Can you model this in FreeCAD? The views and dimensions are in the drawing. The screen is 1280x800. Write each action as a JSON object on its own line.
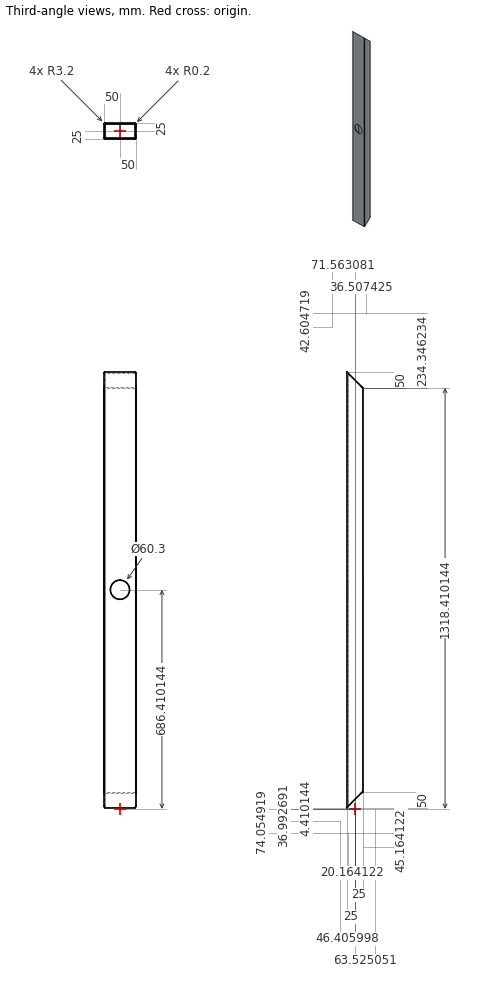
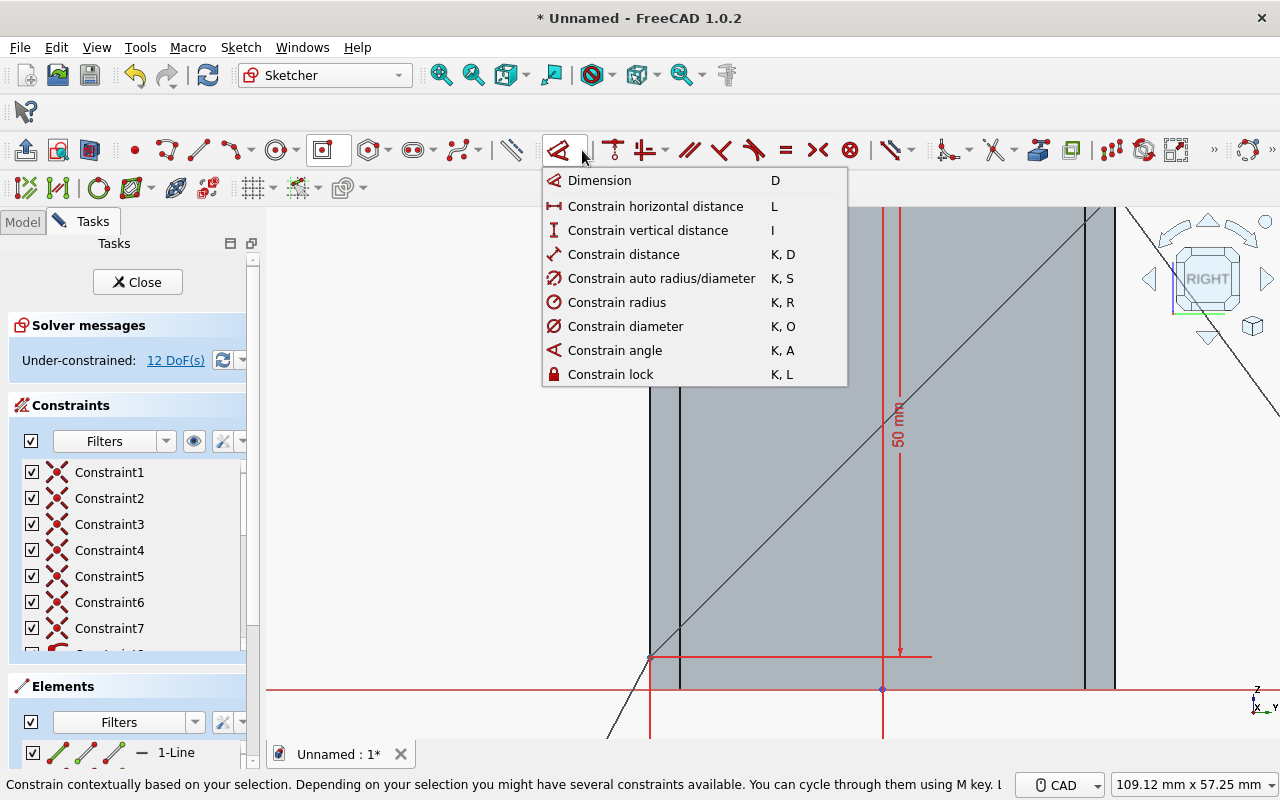
{"action": "left_click", "coordinate": [695, 230]}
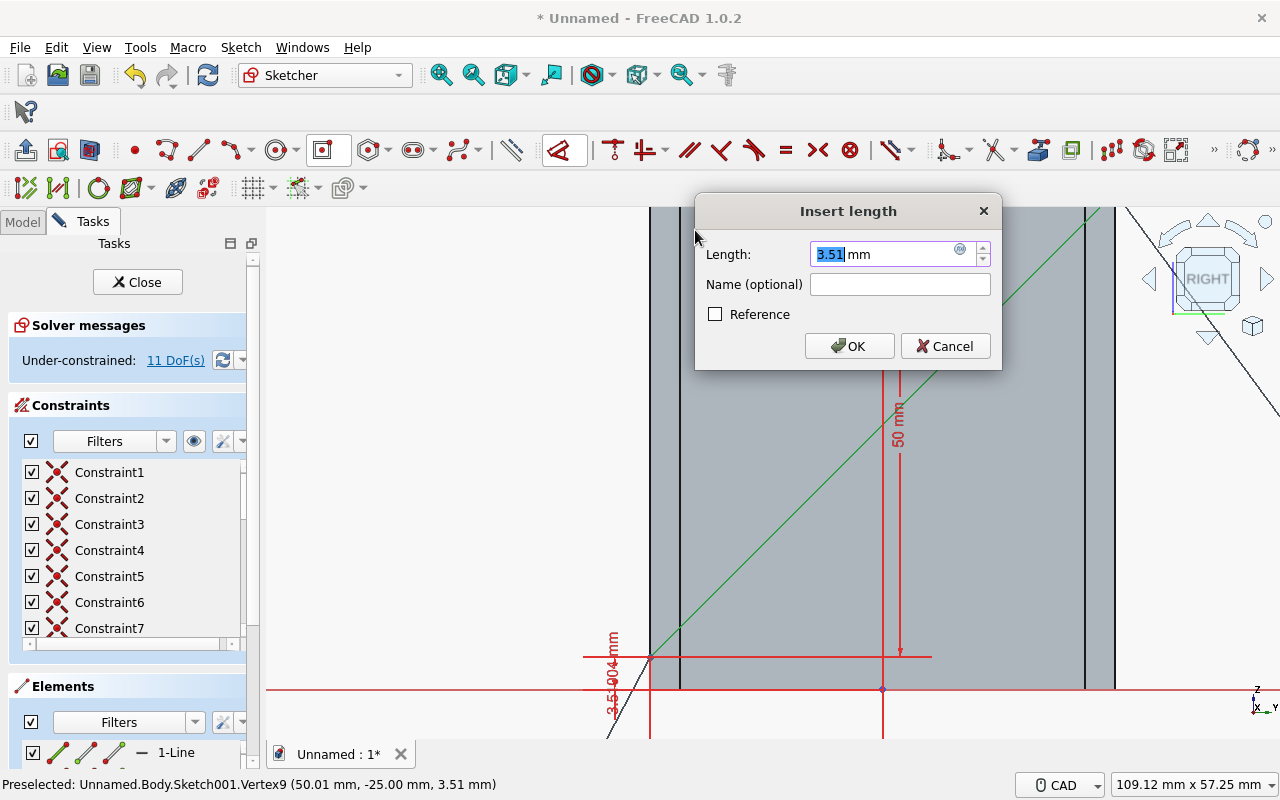
{"action": "type", "text": "4.410144"}
{"action": "key", "text": "Return"}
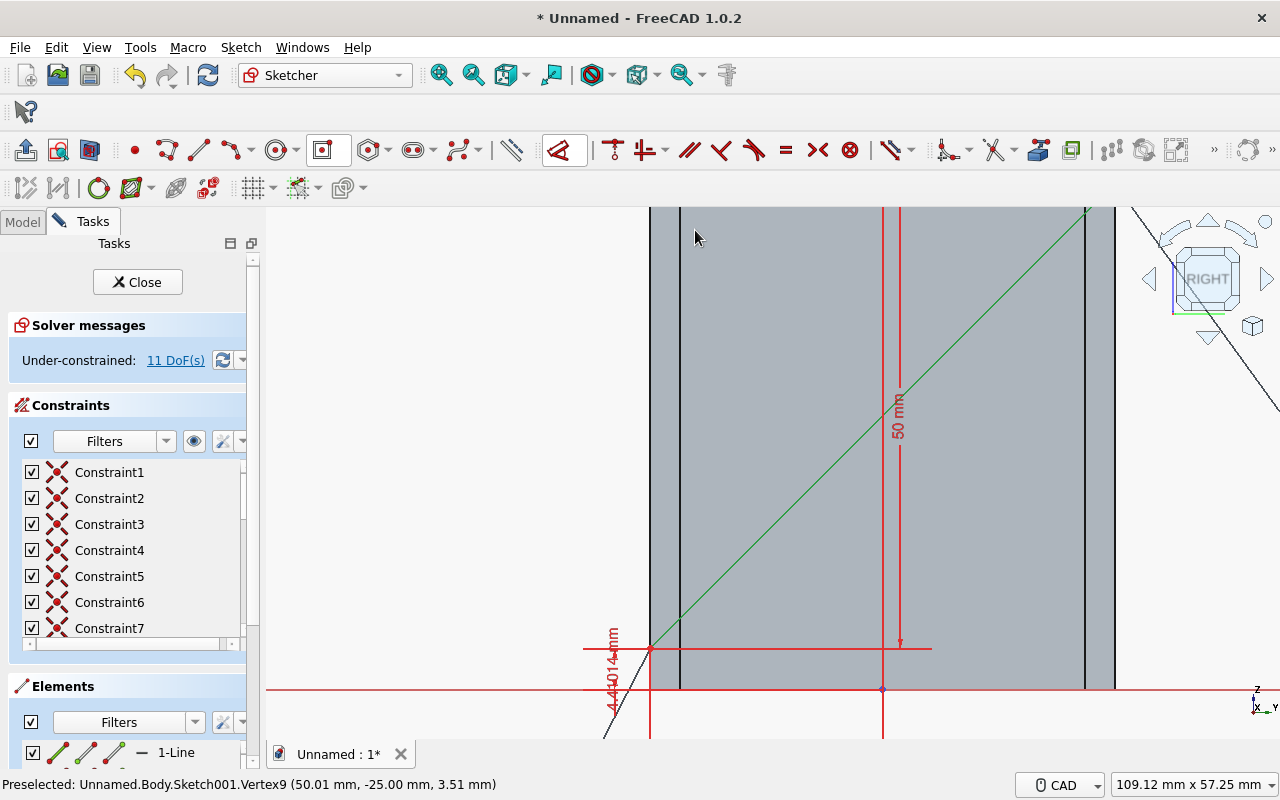
{"action": "scroll", "coordinate": [701, 654], "scroll_direction": "down", "scroll_amount": 18}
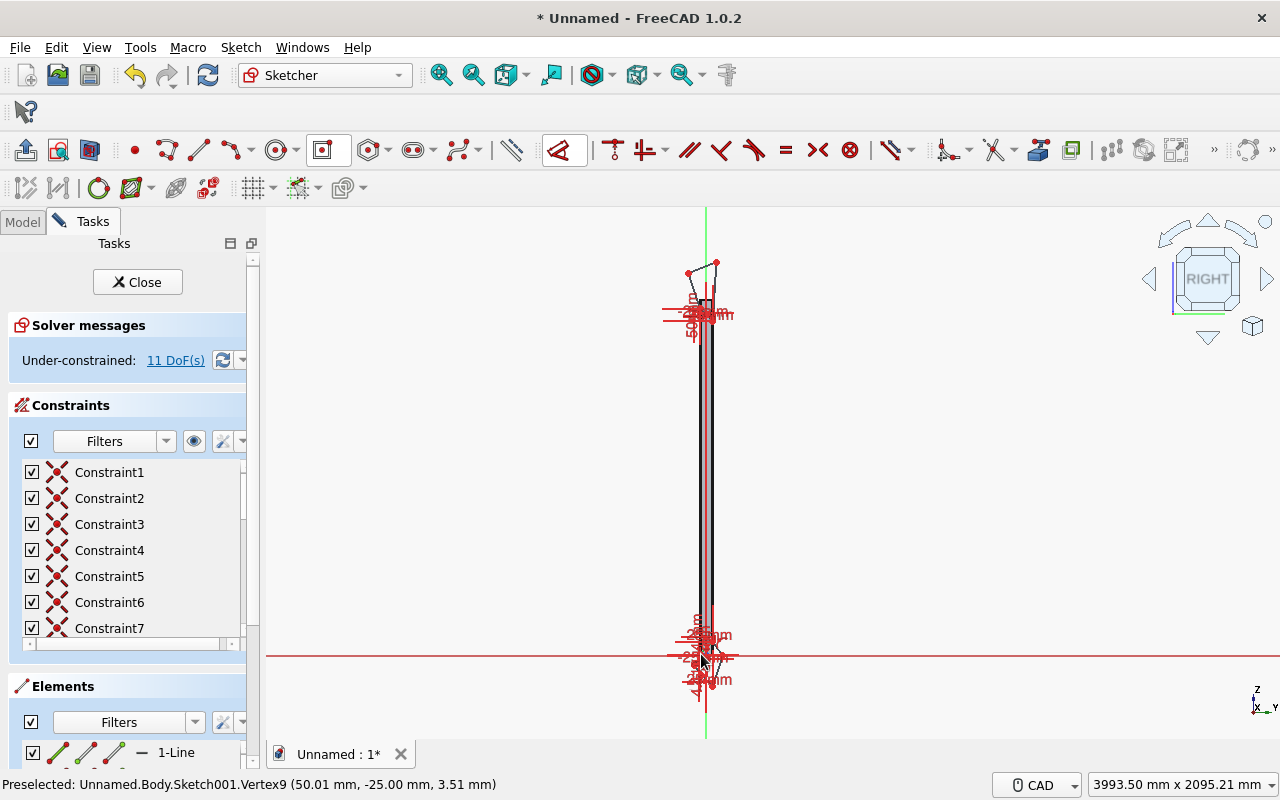
{"action": "scroll", "coordinate": [701, 469], "scroll_direction": "down", "scroll_amount": 1}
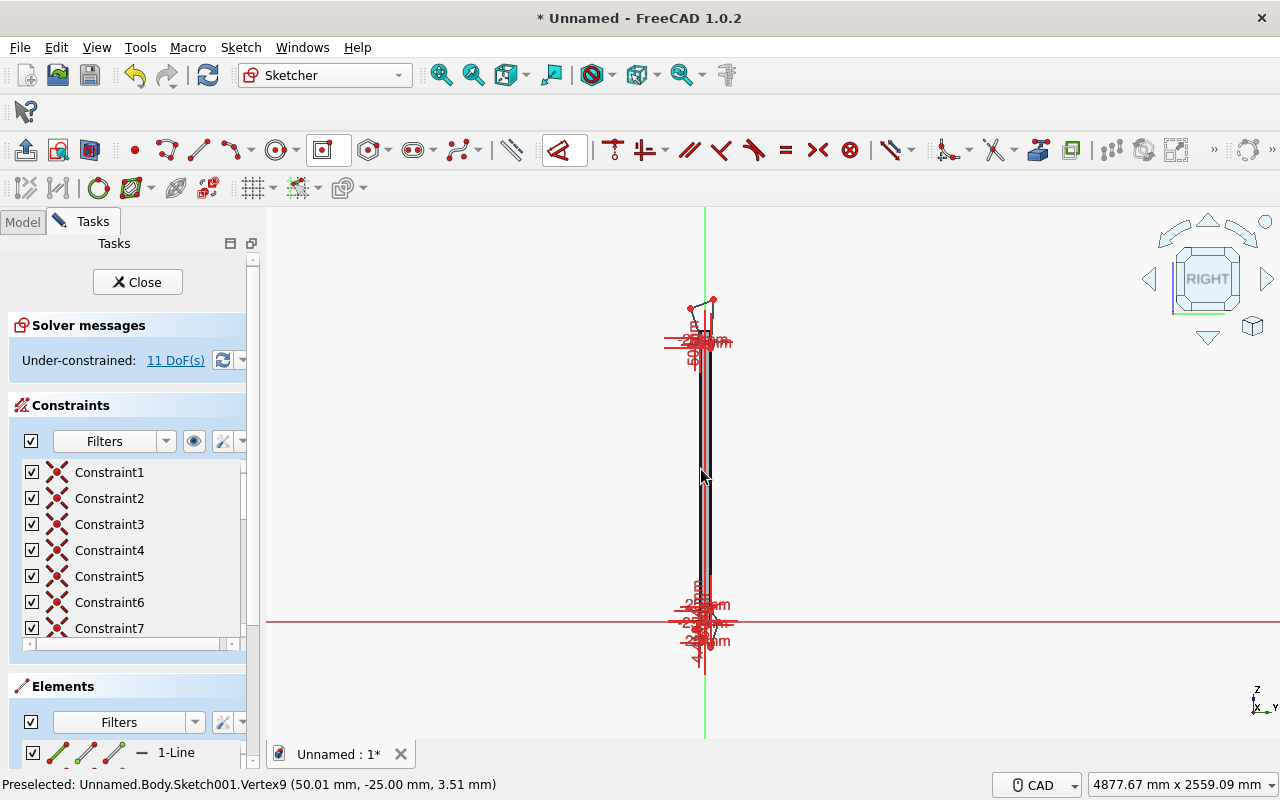
{"action": "scroll", "coordinate": [714, 300], "scroll_direction": "up", "scroll_amount": 9}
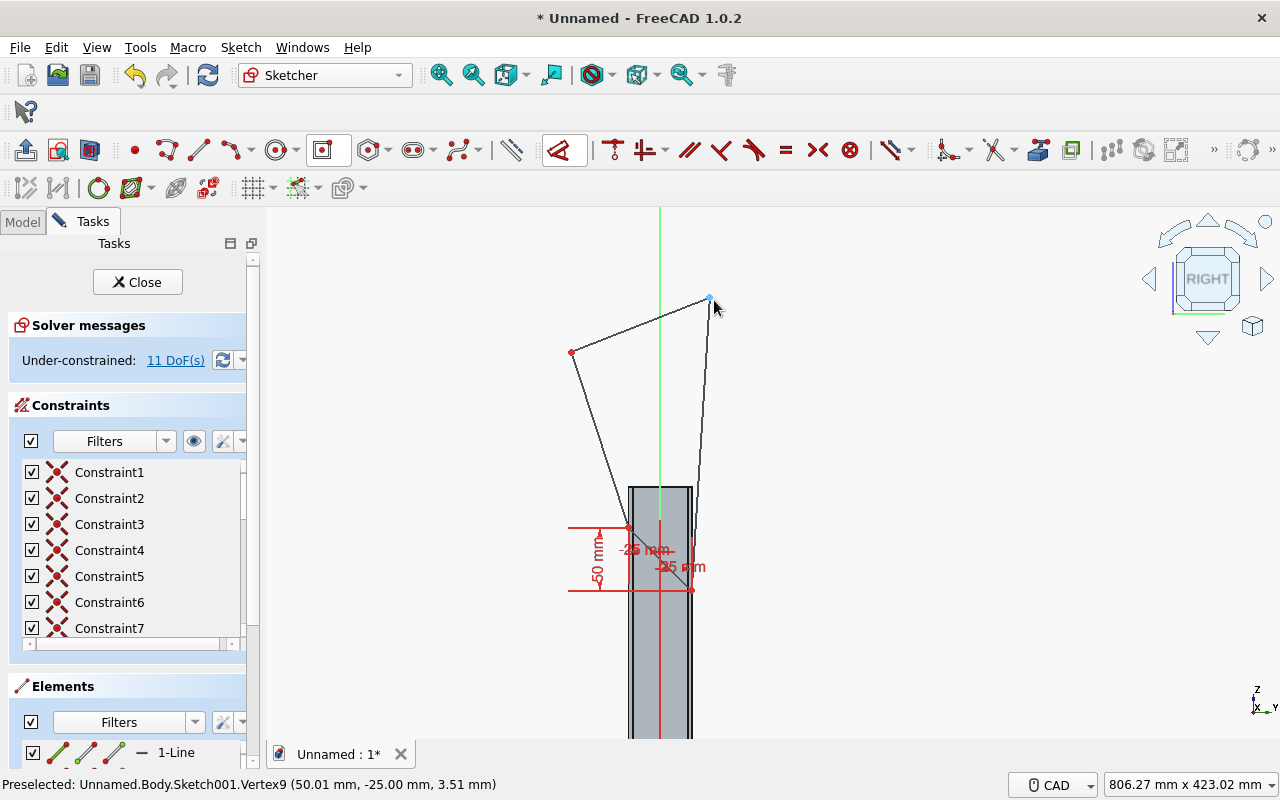
{"action": "left_click", "coordinate": [710, 298]}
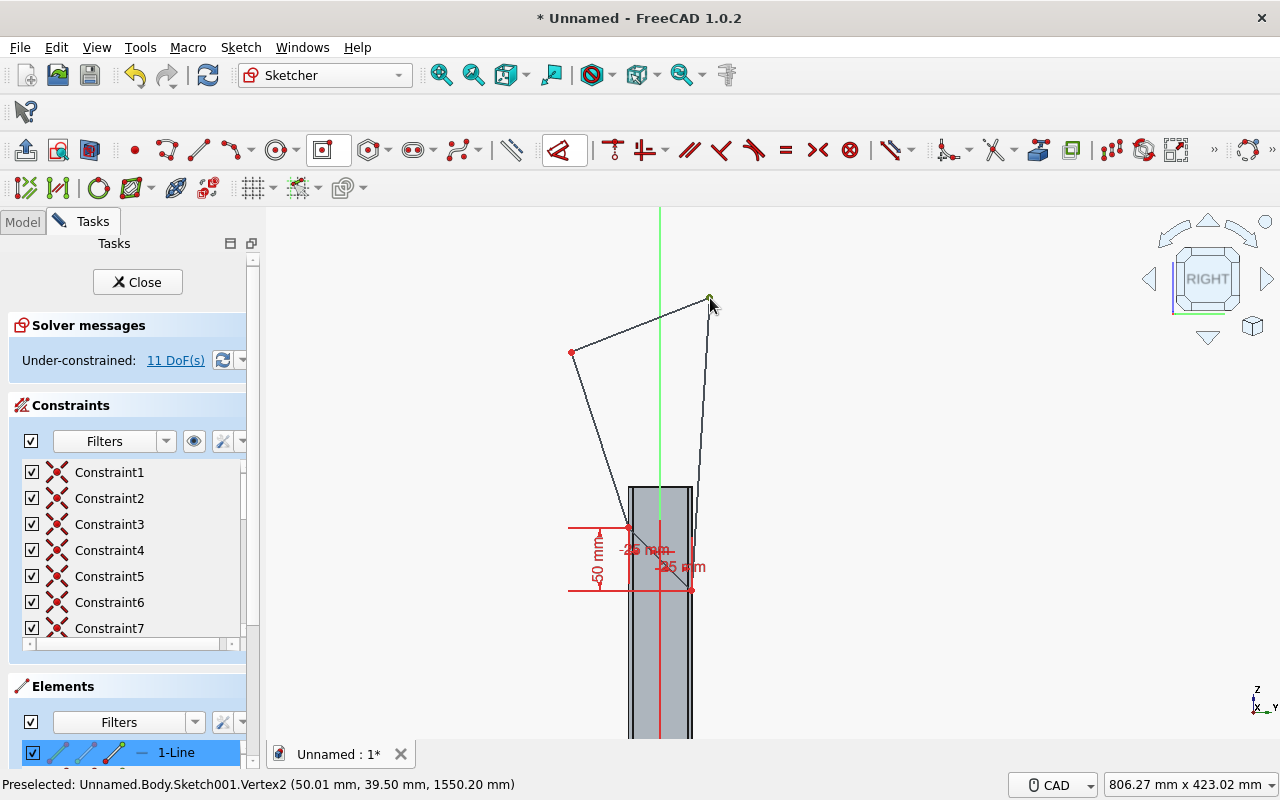
{"action": "left_click", "coordinate": [582, 150]}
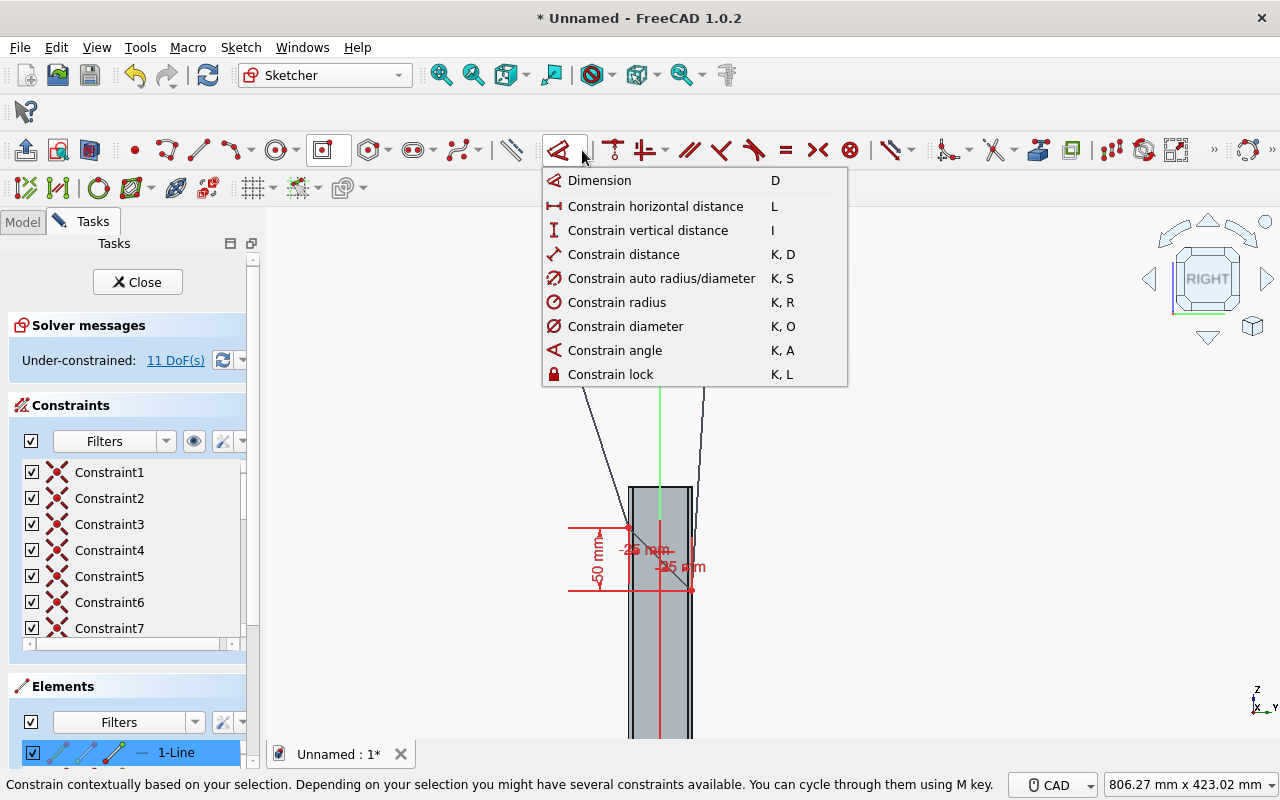
{"action": "left_click", "coordinate": [695, 206]}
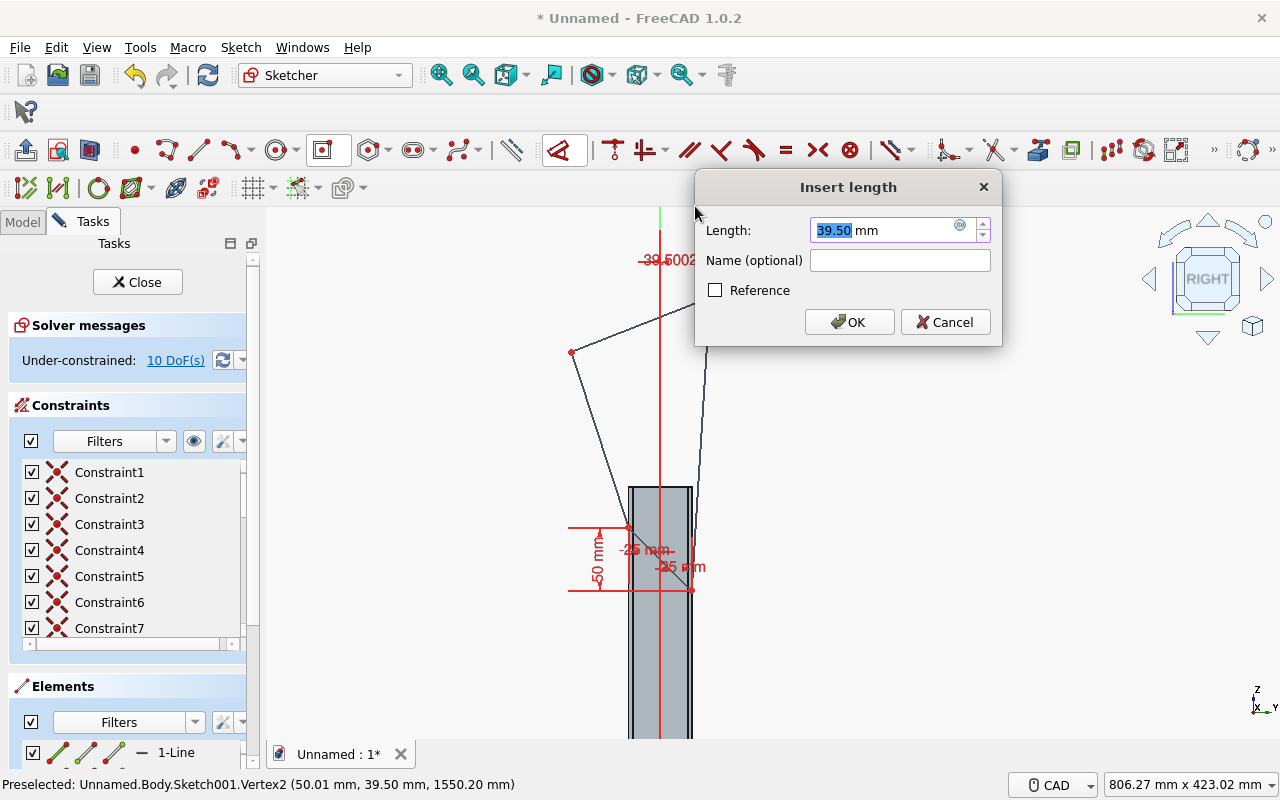
{"action": "type", "text": "36.507425"}
{"action": "key", "text": "Return"}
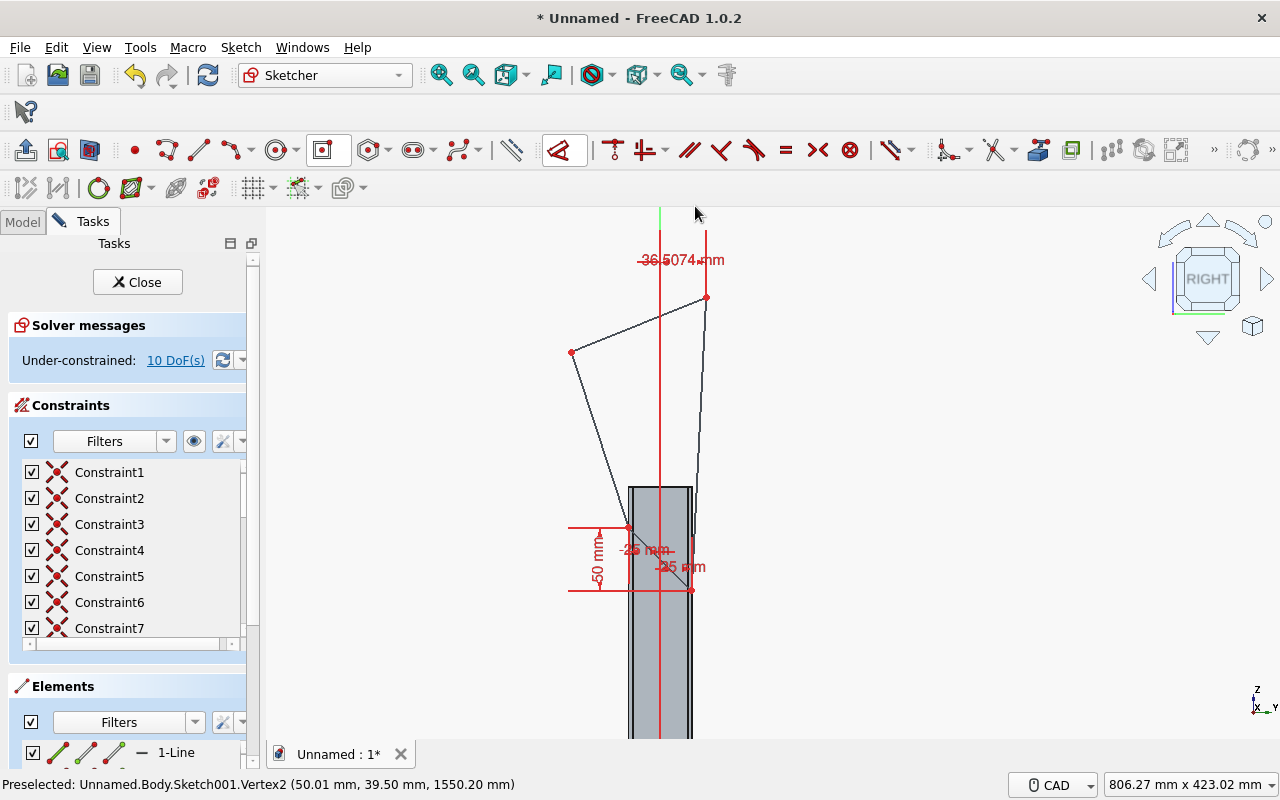
{"action": "left_click", "coordinate": [571, 352]}